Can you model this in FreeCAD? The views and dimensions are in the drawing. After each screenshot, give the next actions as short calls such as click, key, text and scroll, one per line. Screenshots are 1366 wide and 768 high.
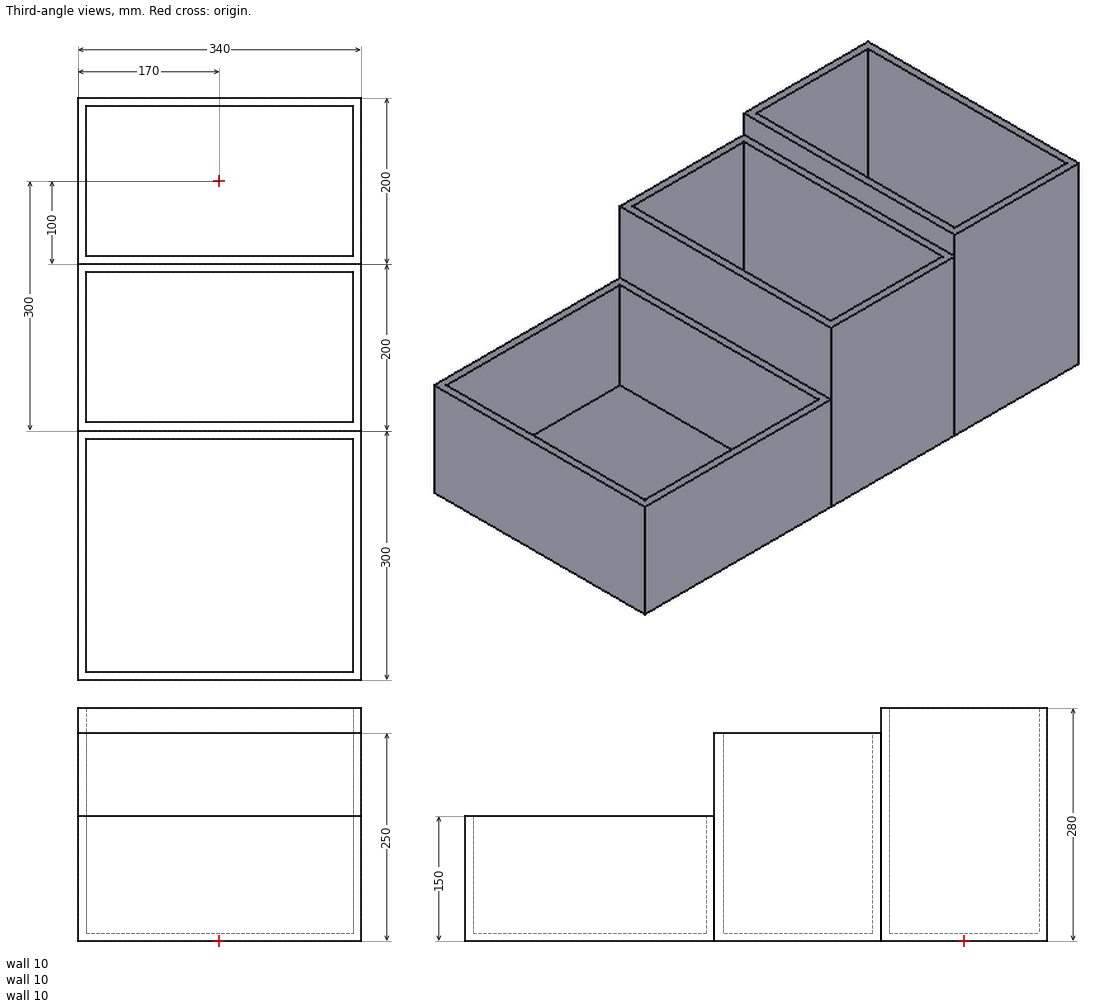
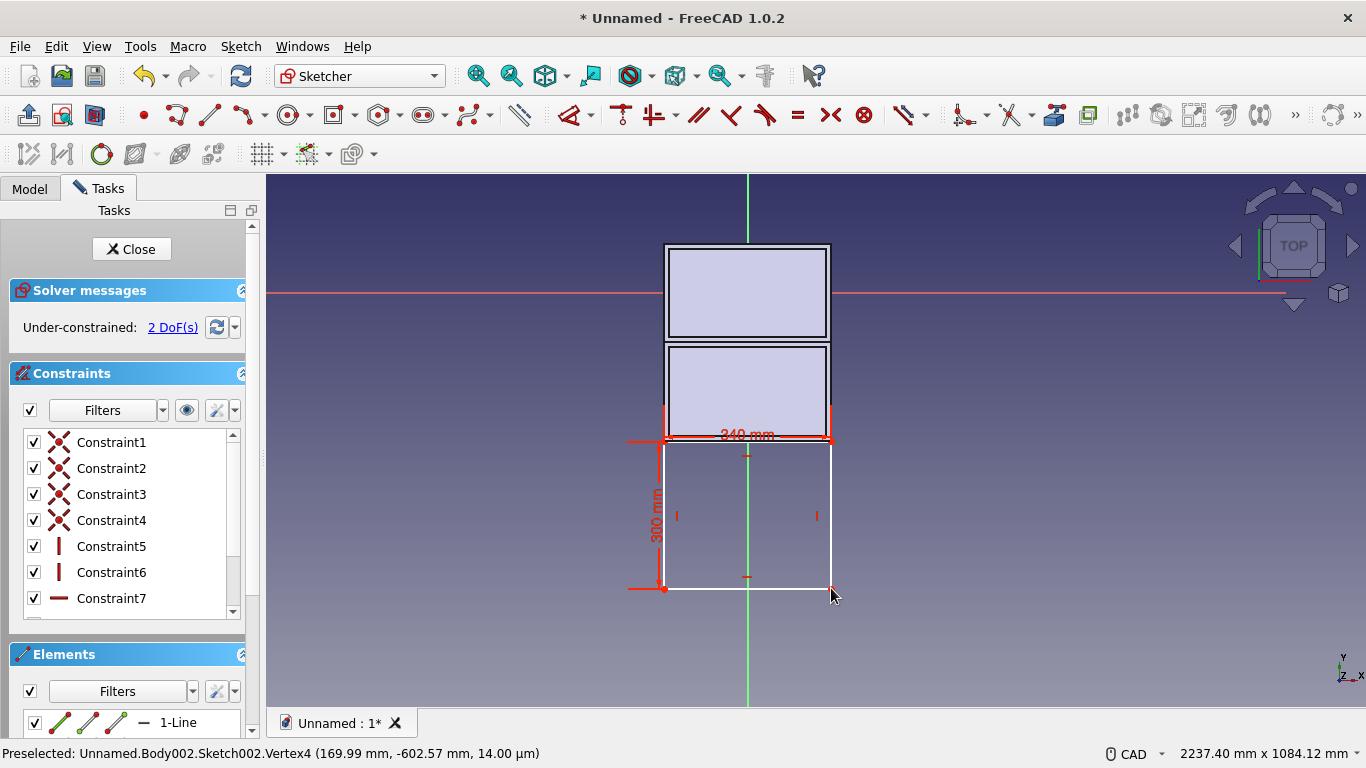
key(d)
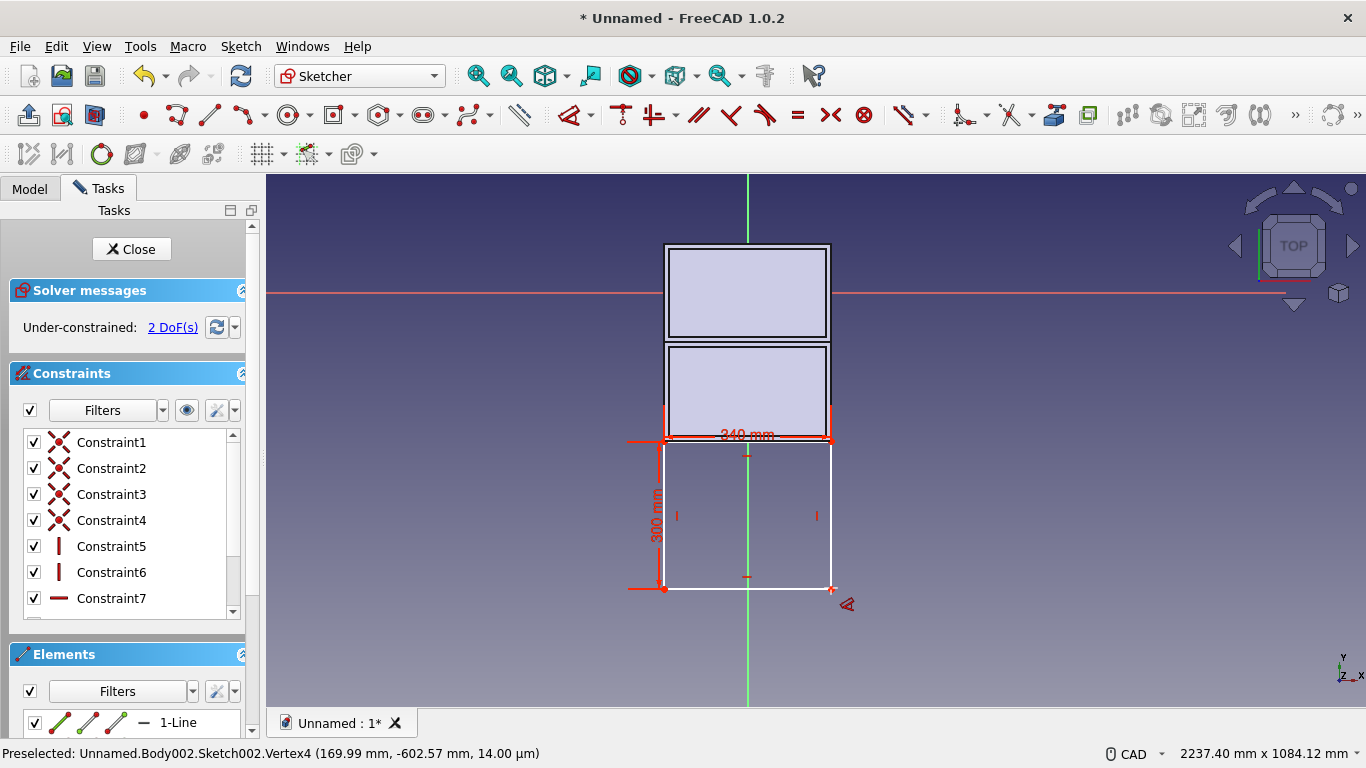
click(664, 442)
click(706, 259)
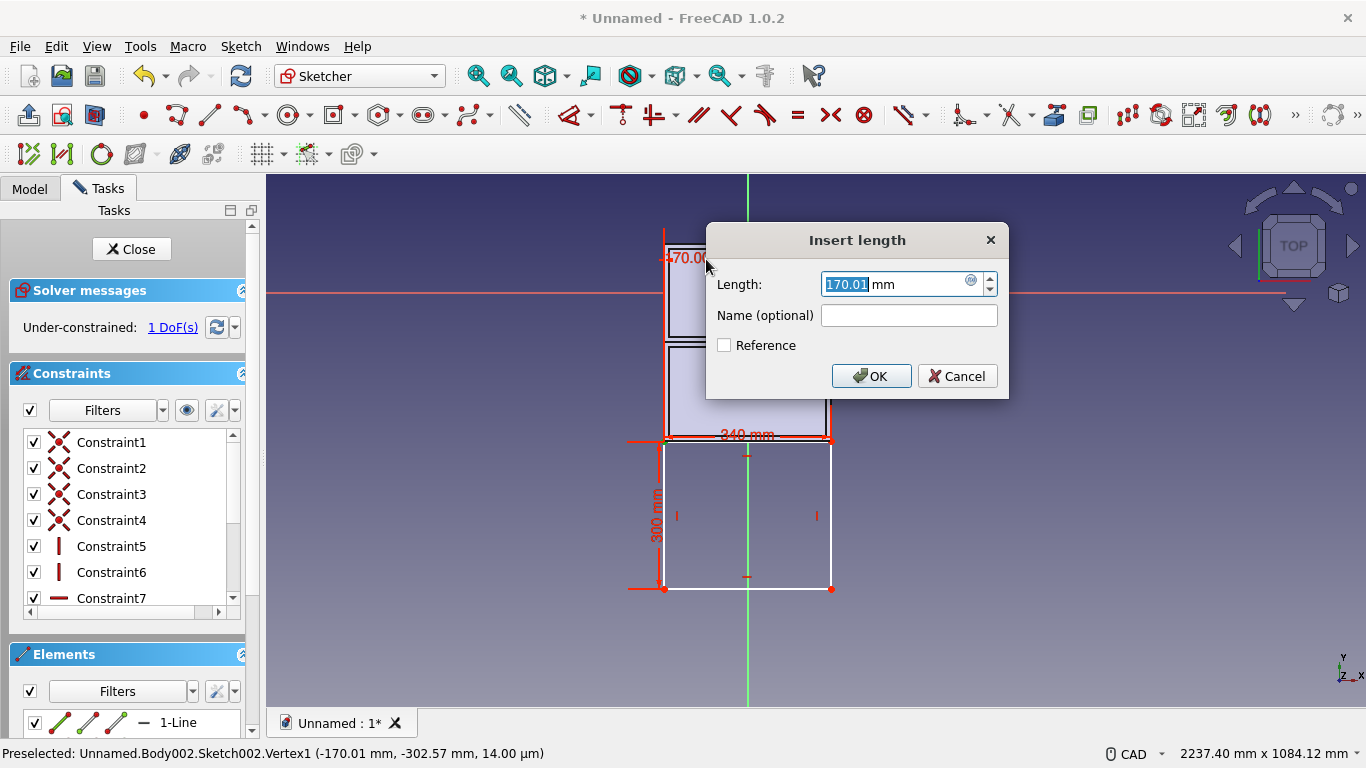
text(170)
key(Return)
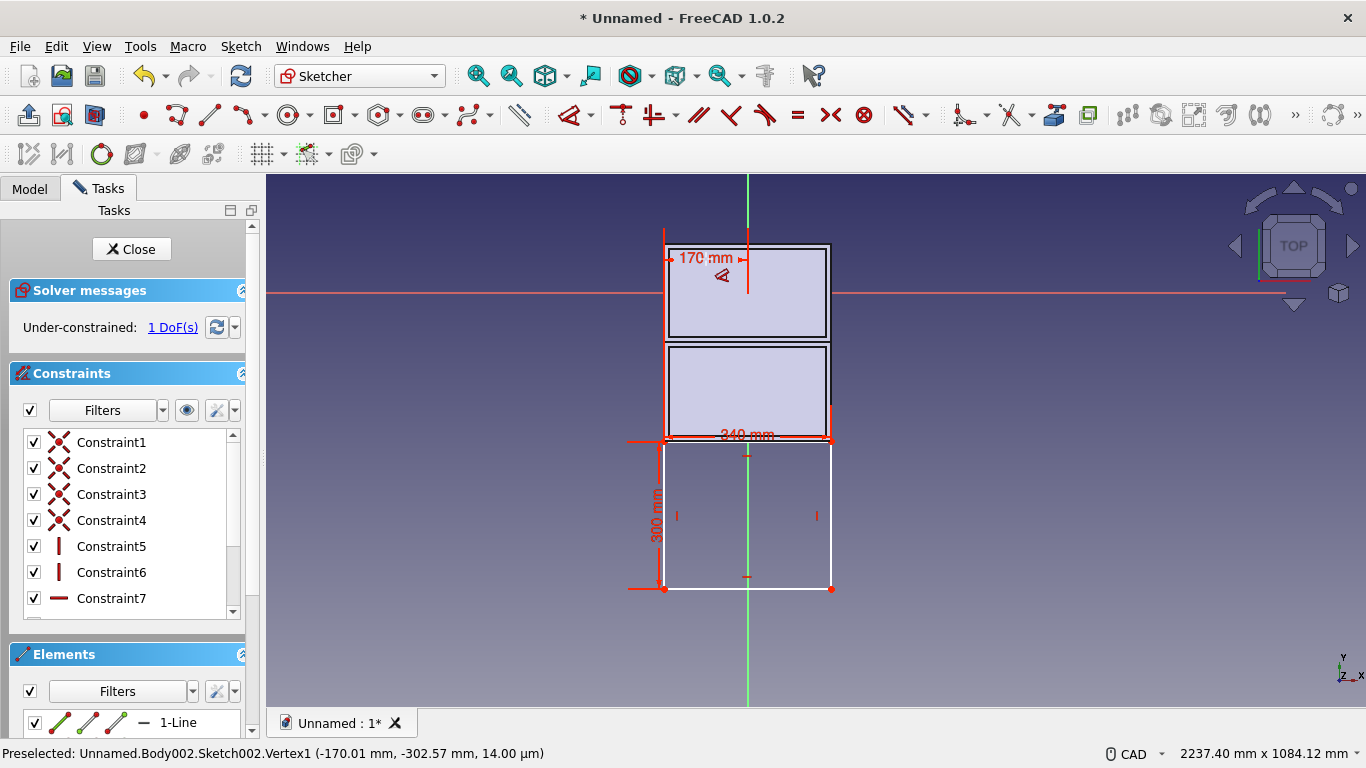
click(664, 442)
click(630, 368)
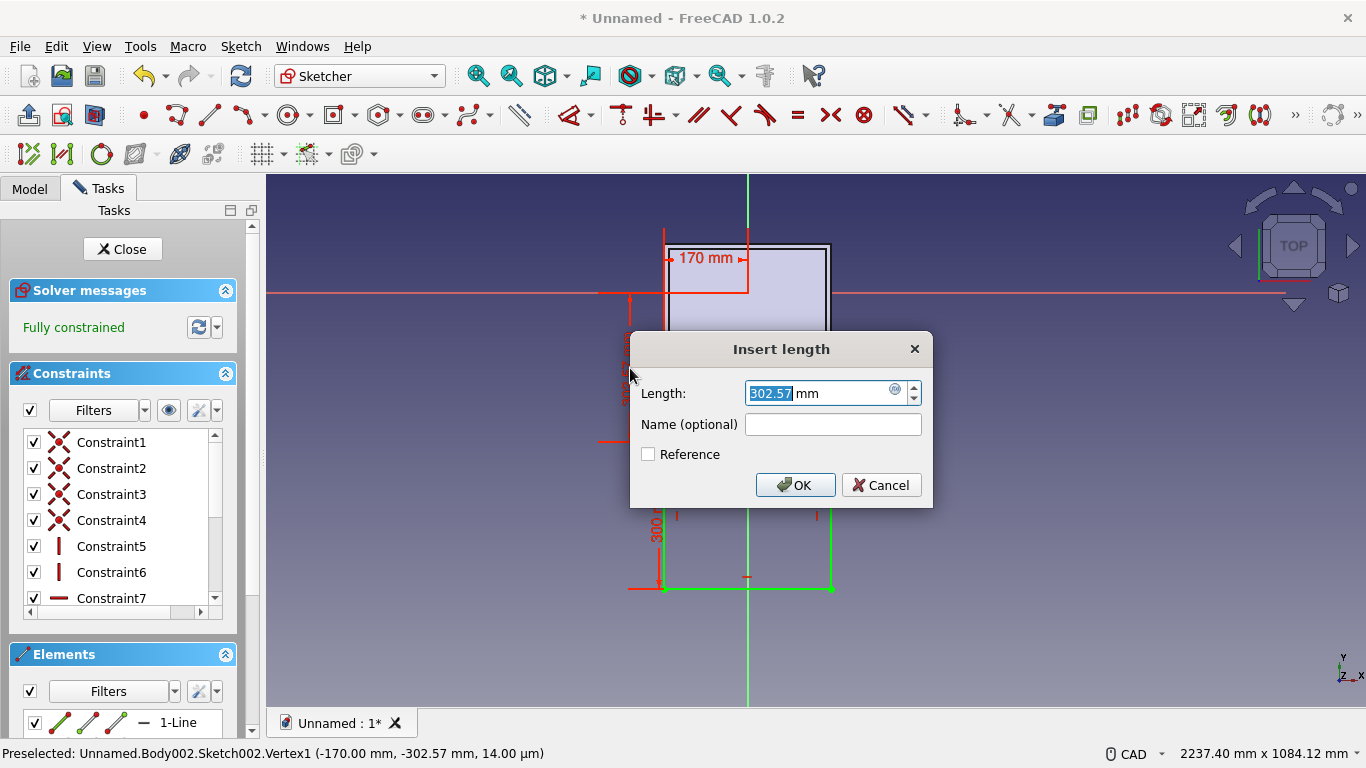
text(300)
key(Return)
key(Escape)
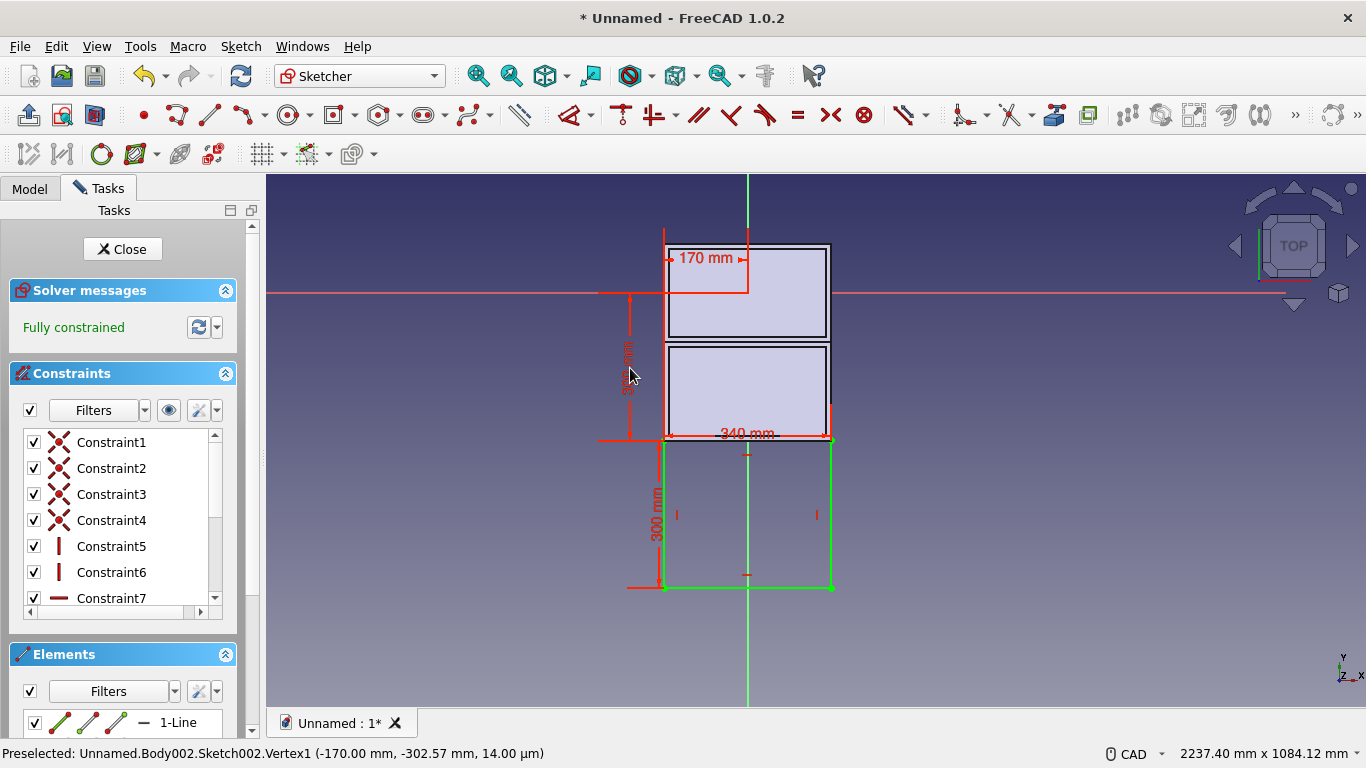
click(123, 249)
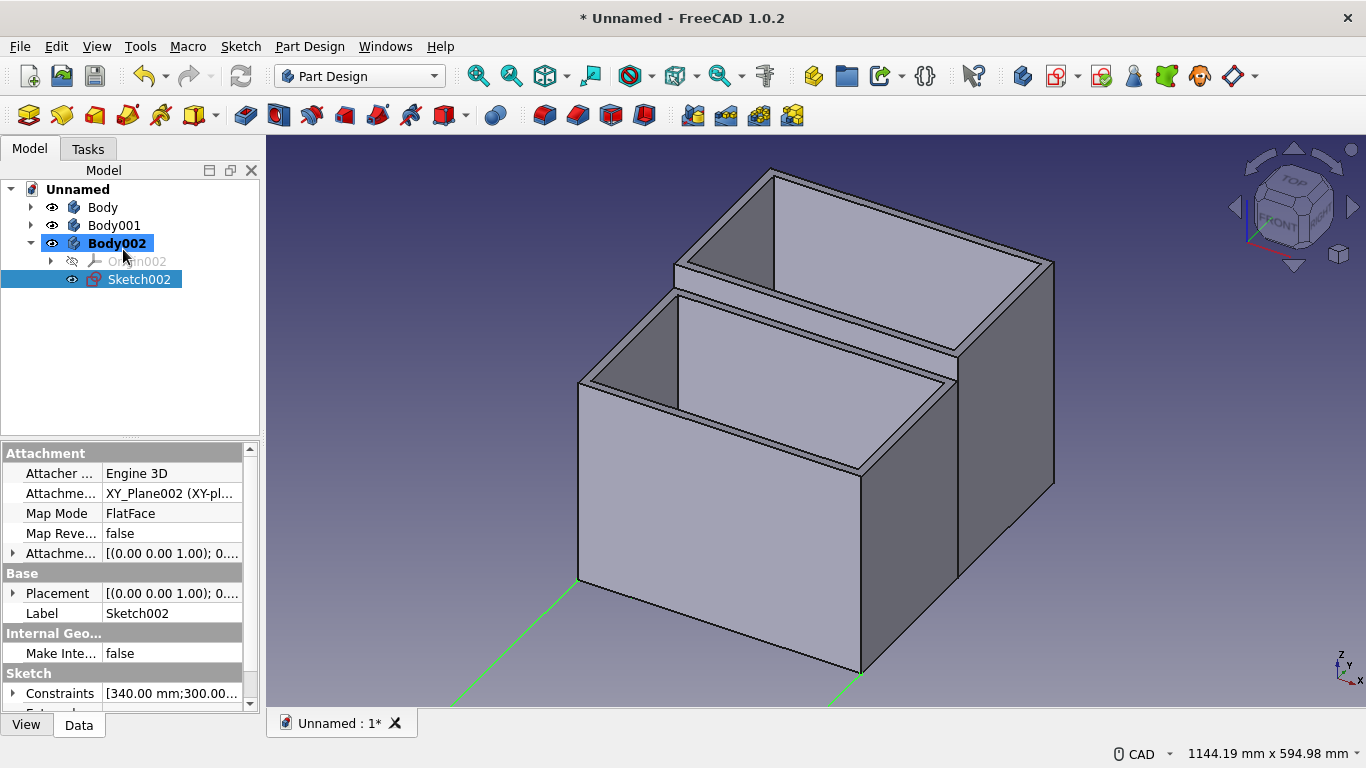
click(29, 116)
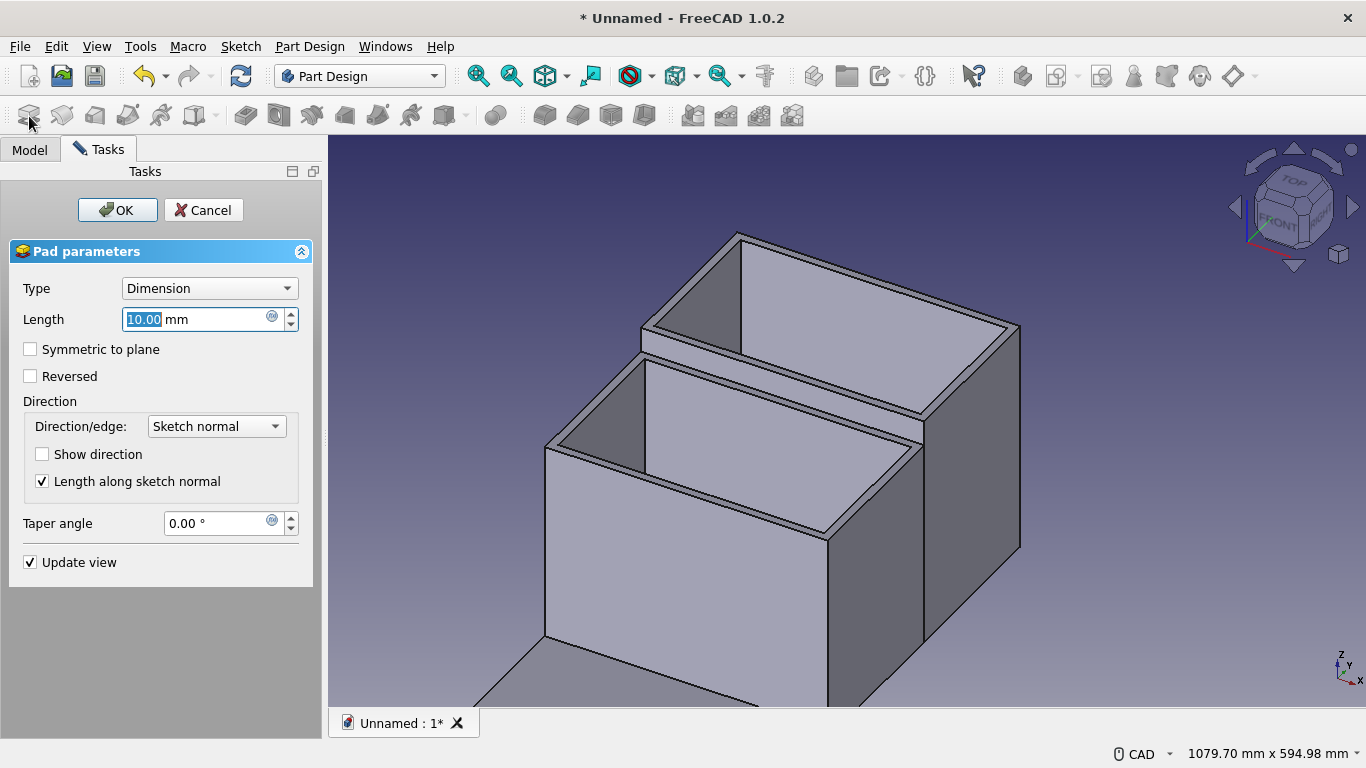
text(150)
key(Tab)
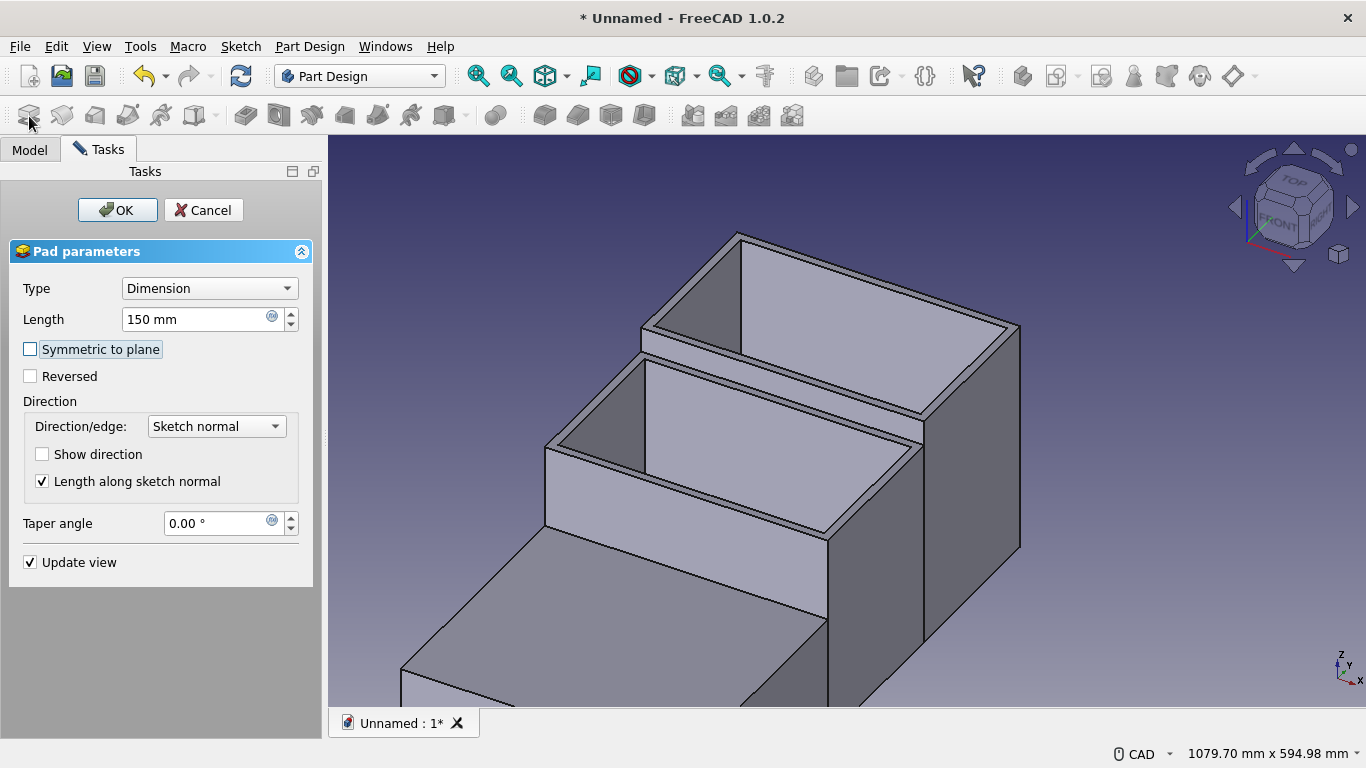
click(118, 210)